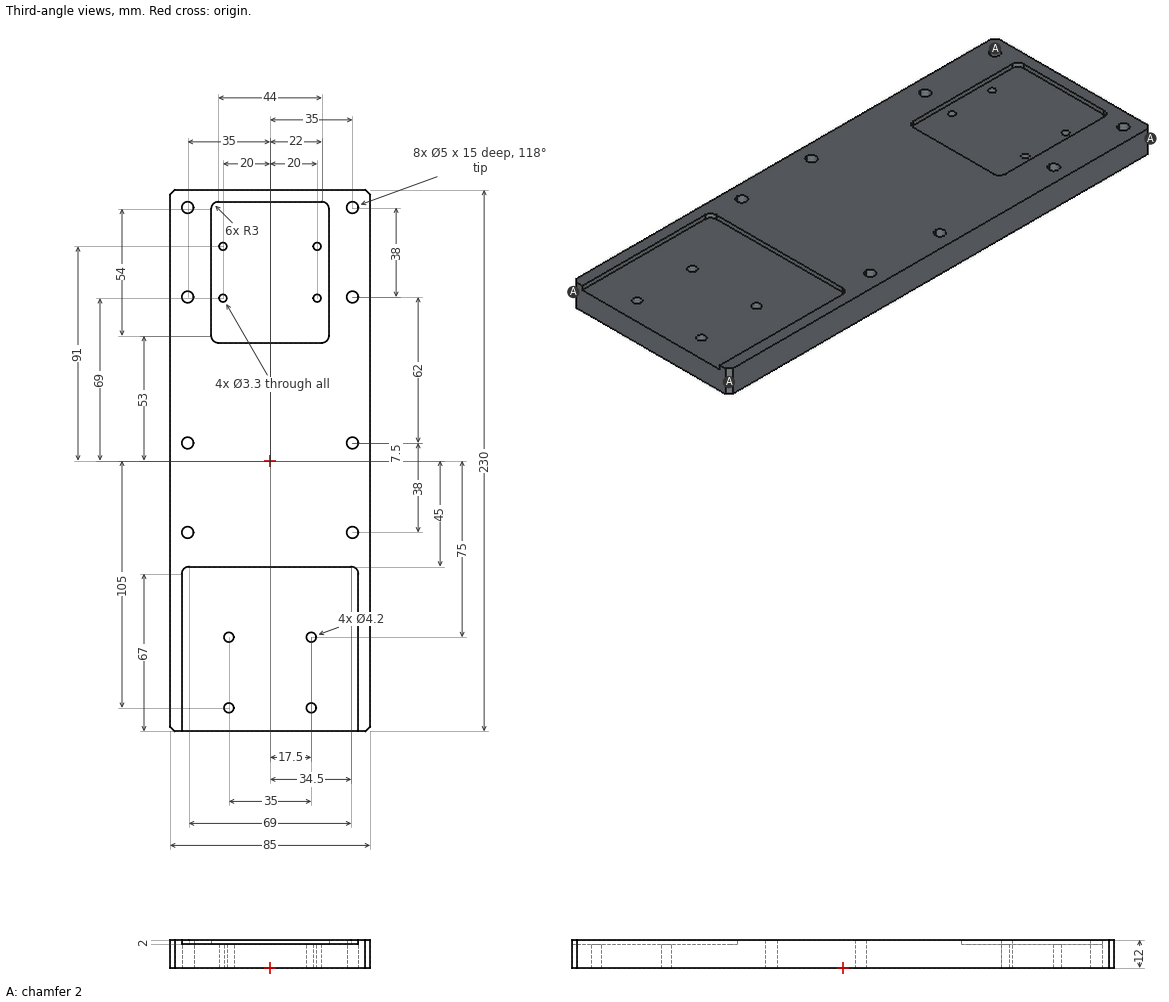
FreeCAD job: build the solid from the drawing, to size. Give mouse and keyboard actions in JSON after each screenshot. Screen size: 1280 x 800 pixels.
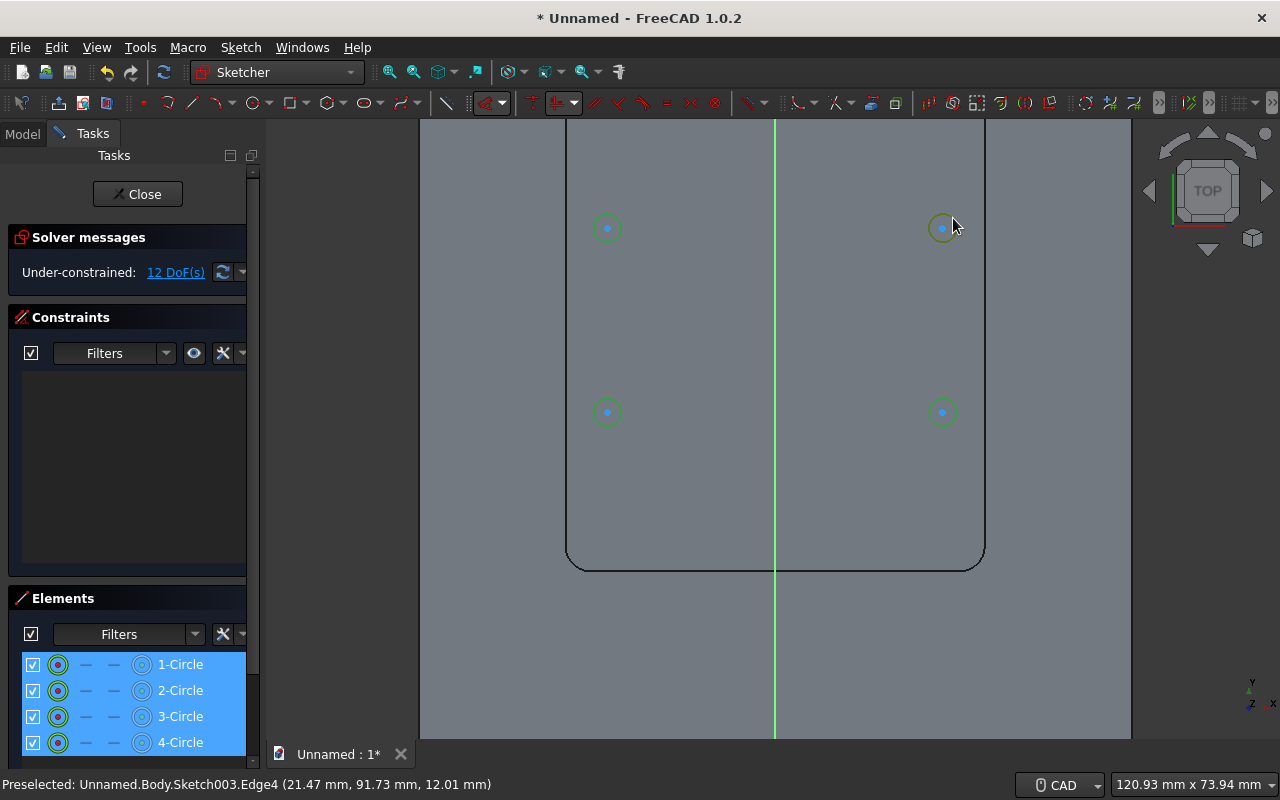
{"action": "key", "text": "e"}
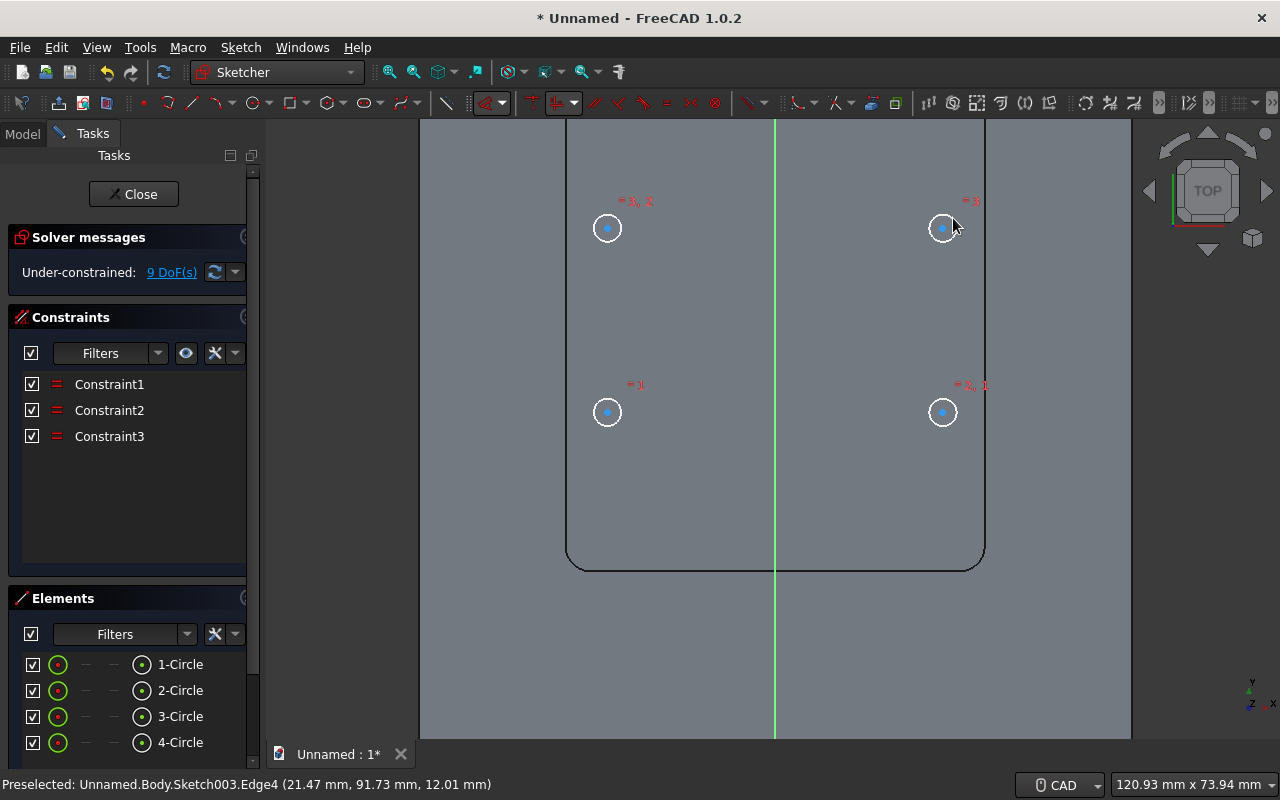
{"action": "left_click", "coordinate": [607, 412]}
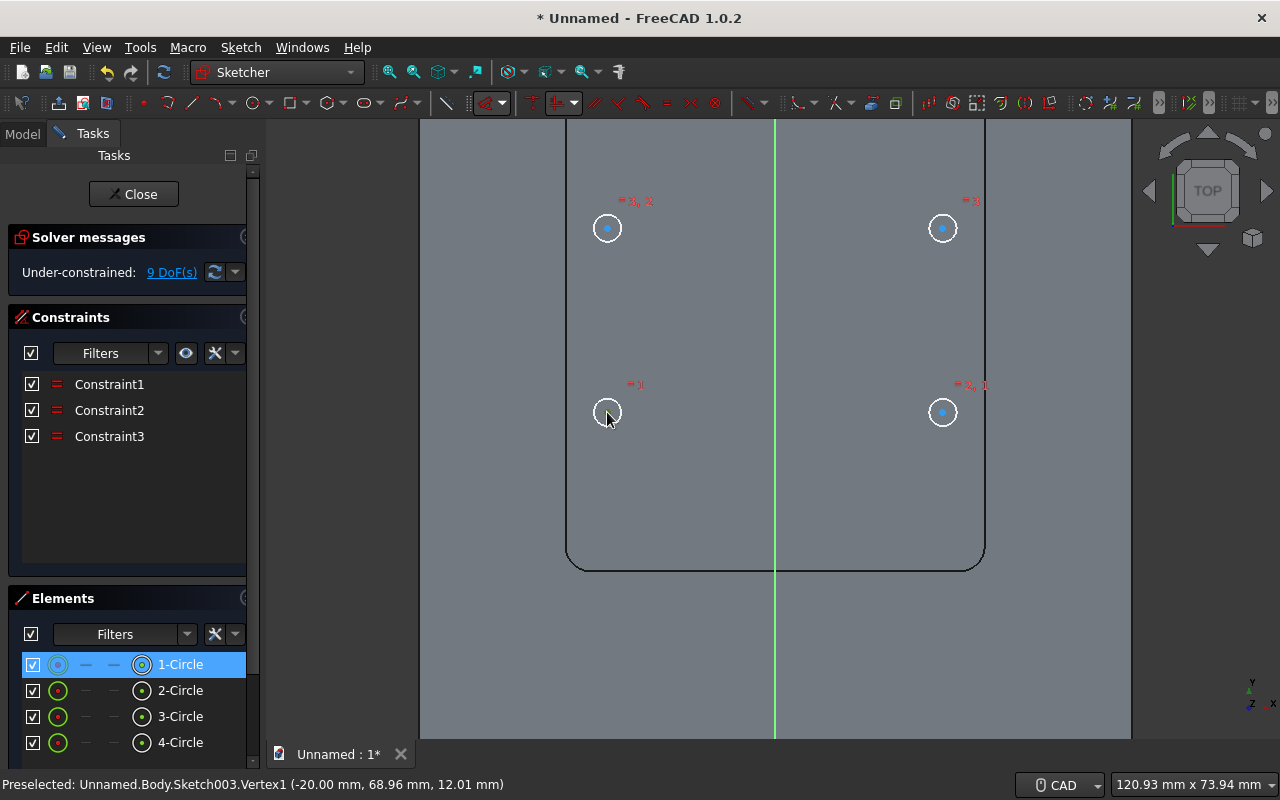
{"action": "left_click", "coordinate": [943, 412]}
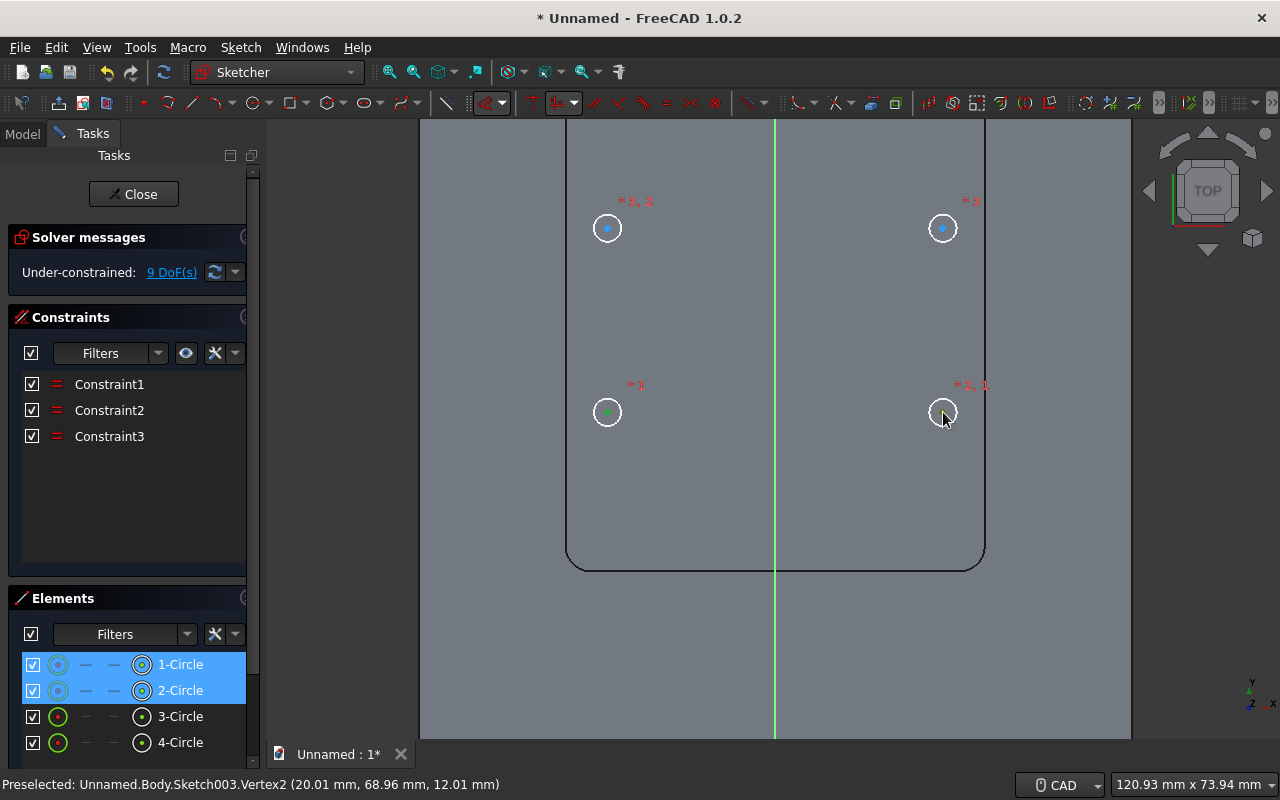
{"action": "key", "text": "h"}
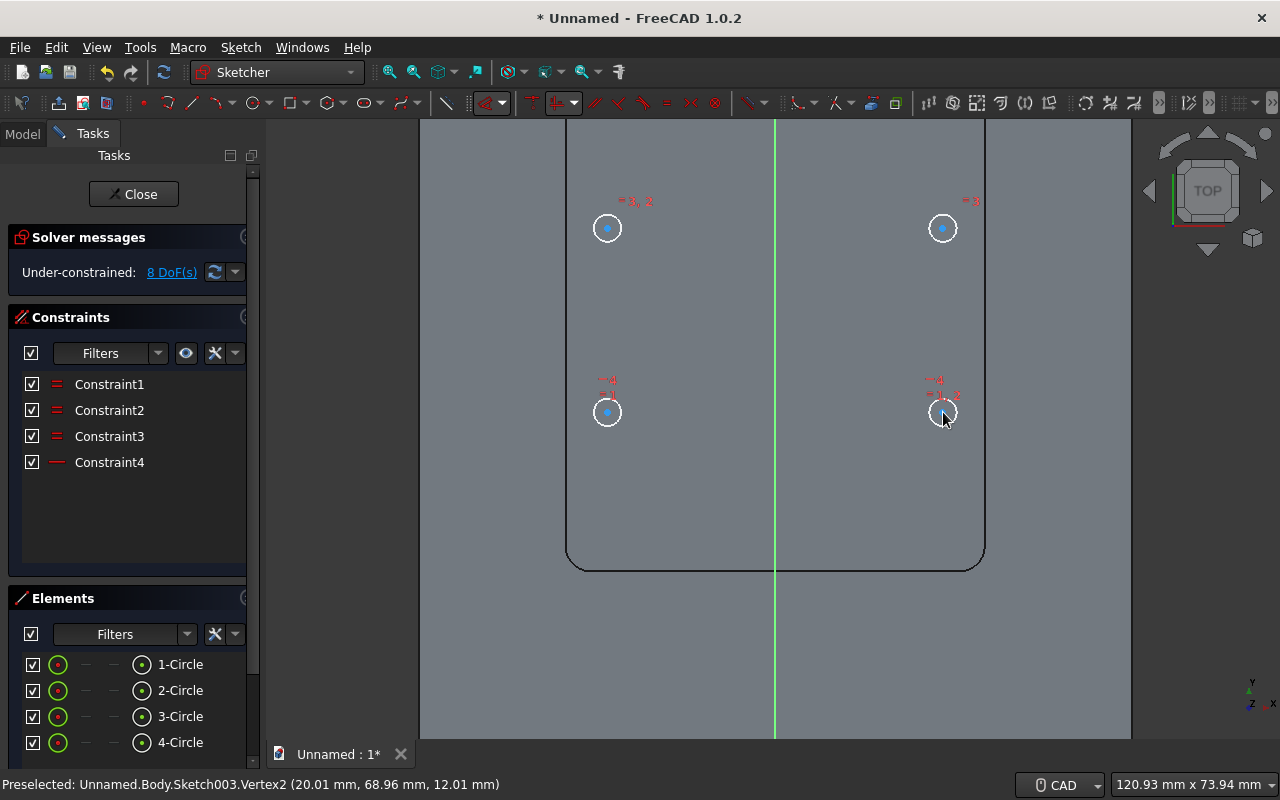
{"action": "left_click", "coordinate": [607, 412]}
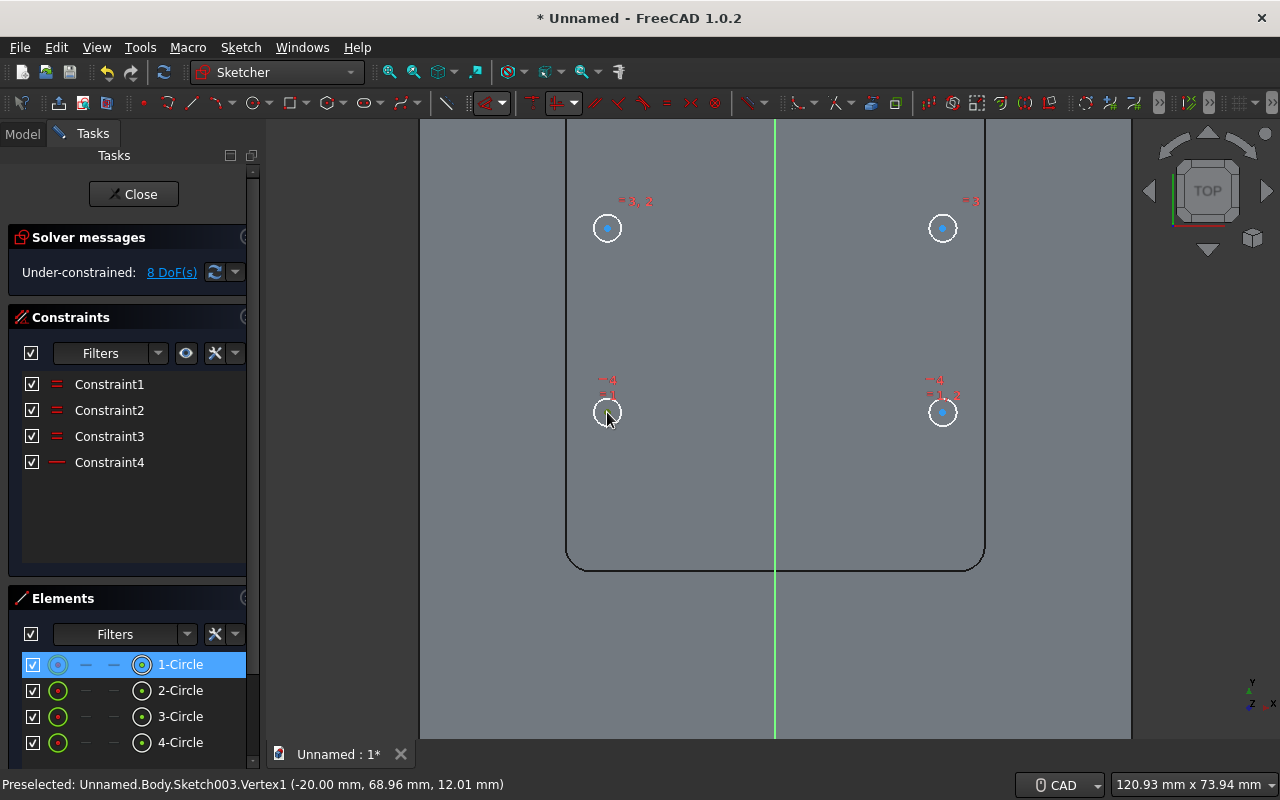
{"action": "left_click", "coordinate": [607, 228]}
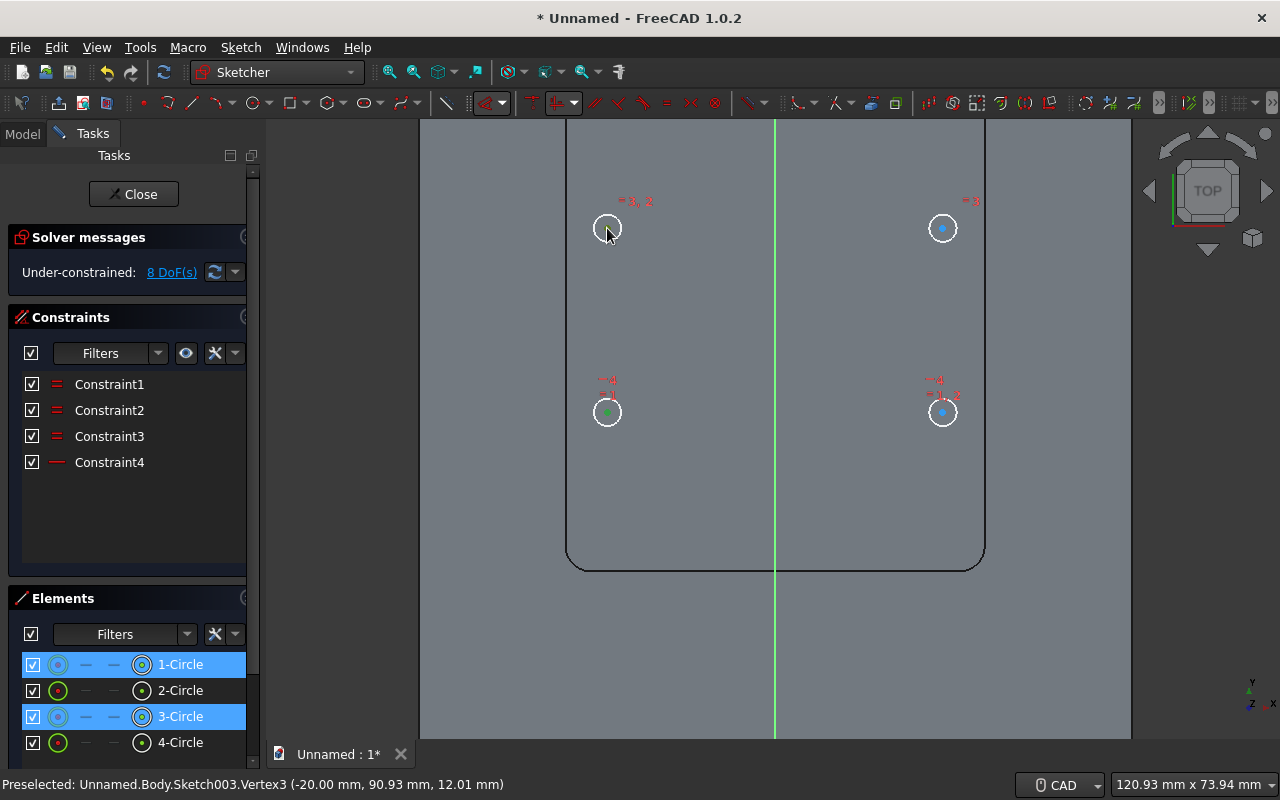
{"action": "key", "text": "v"}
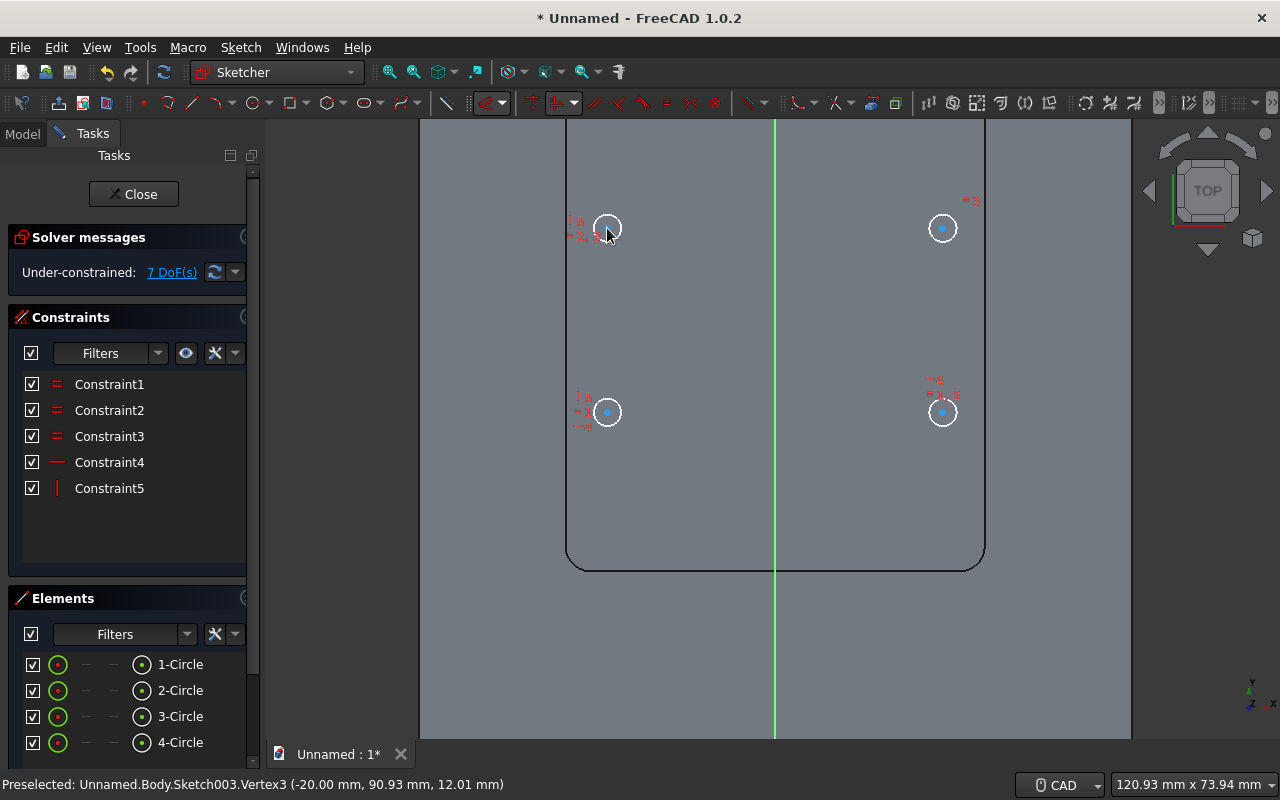
{"action": "left_click", "coordinate": [943, 412]}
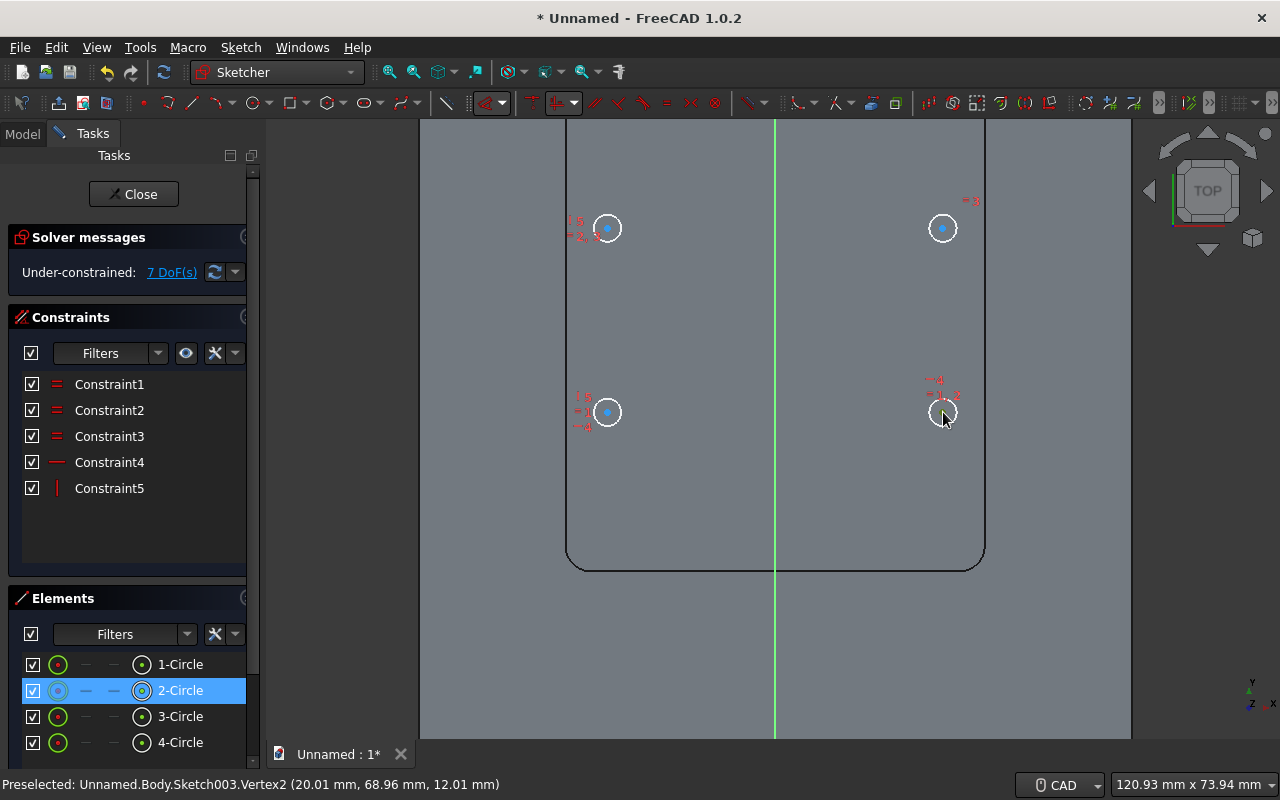
{"action": "left_click", "coordinate": [943, 228]}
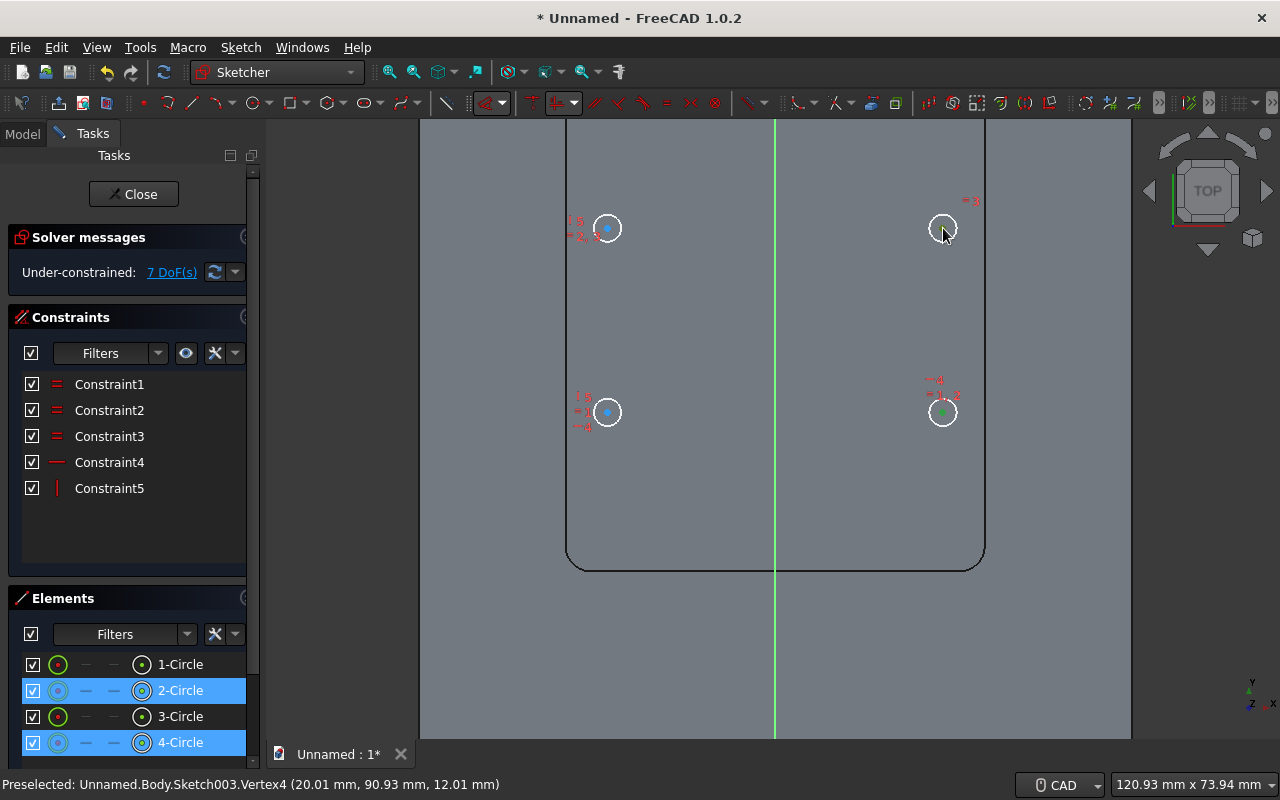
{"action": "key", "text": "v"}